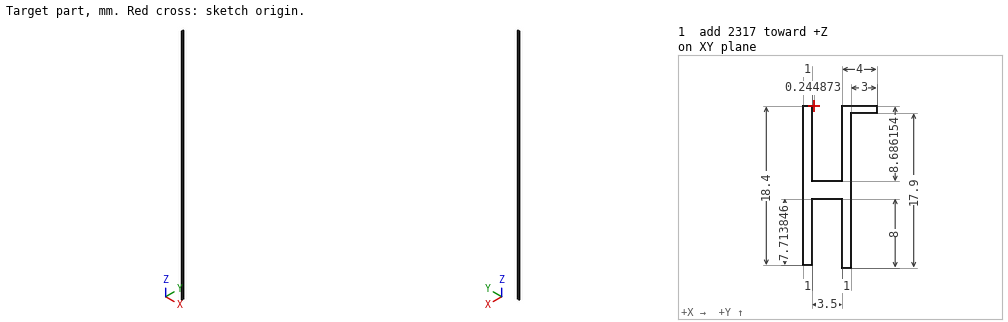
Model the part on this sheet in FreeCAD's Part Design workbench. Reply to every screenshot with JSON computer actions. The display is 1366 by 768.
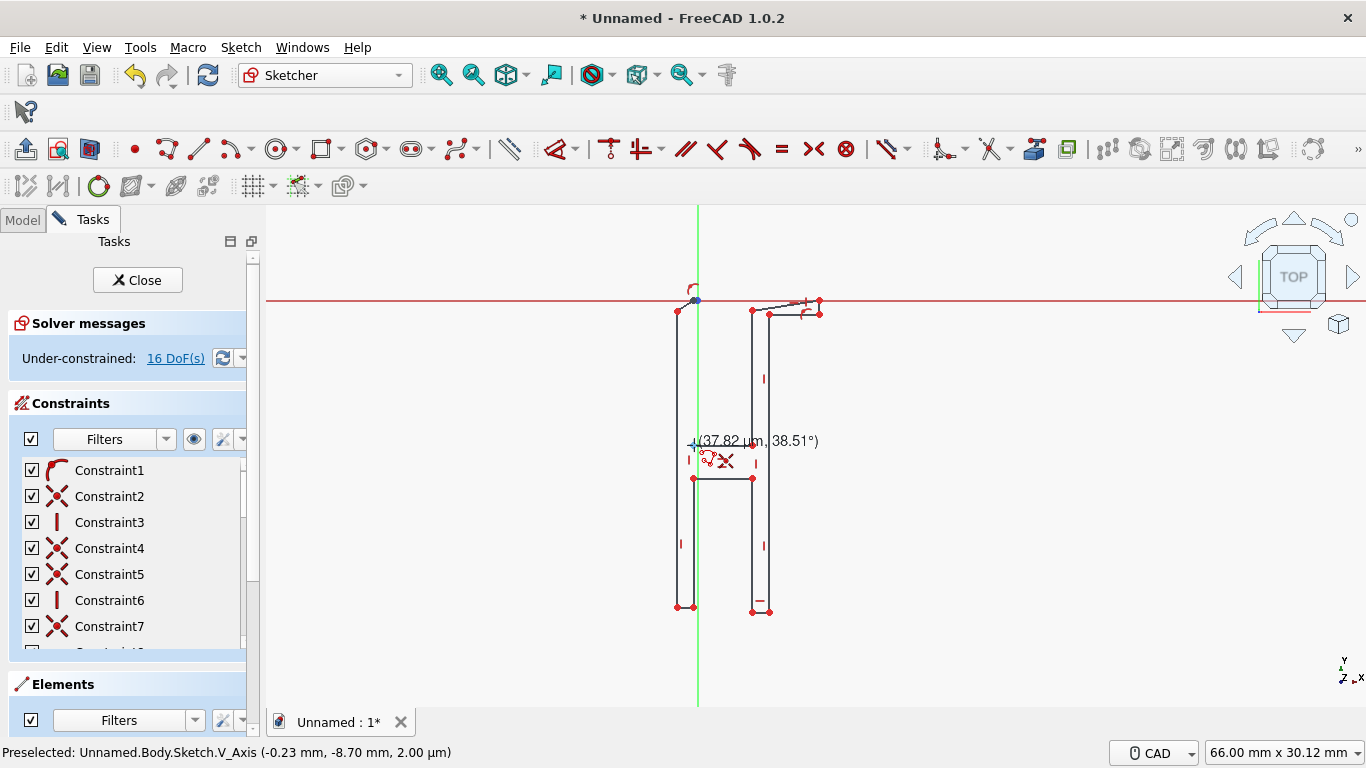
{"action": "scroll", "coordinate": [694, 301], "scroll_direction": "up", "scroll_amount": 7}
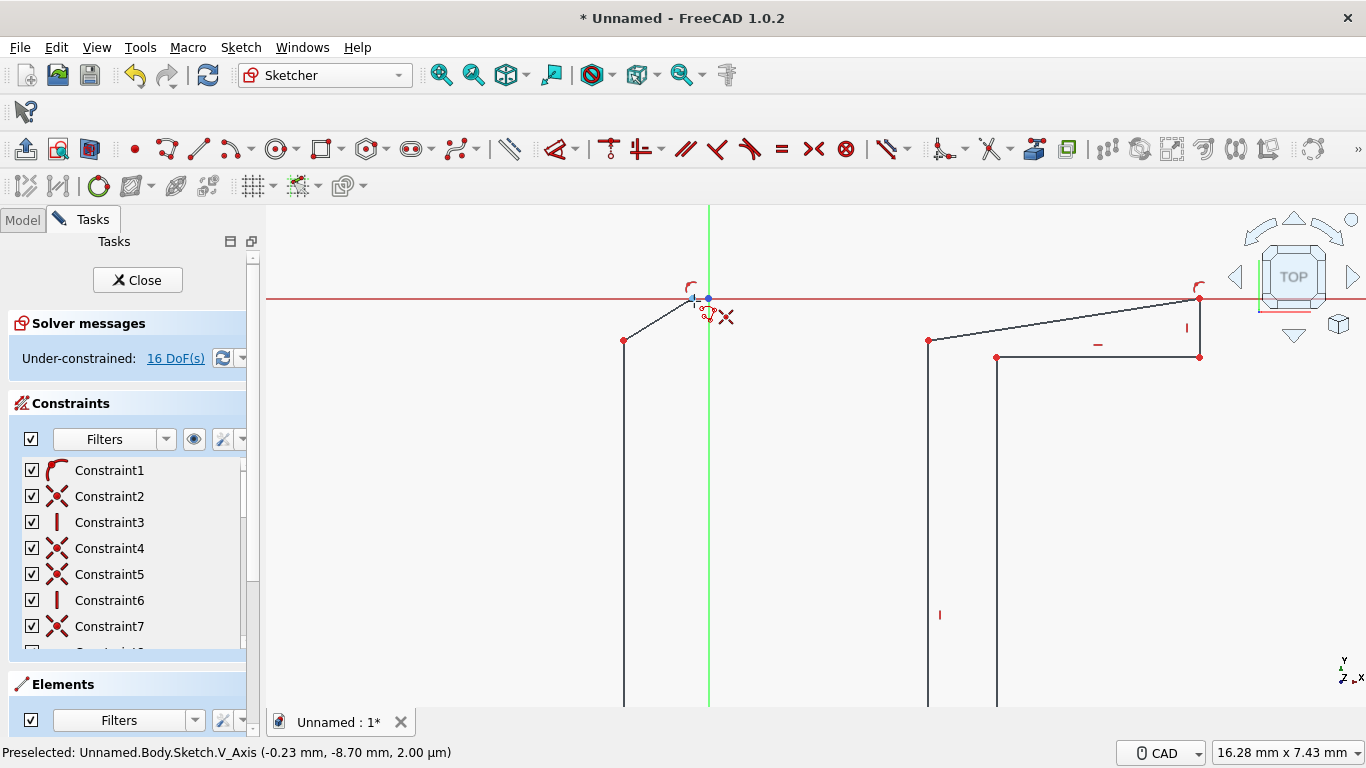
{"action": "left_click", "coordinate": [692, 299]}
{"action": "key", "text": "Escape"}
{"action": "key", "text": "Escape"}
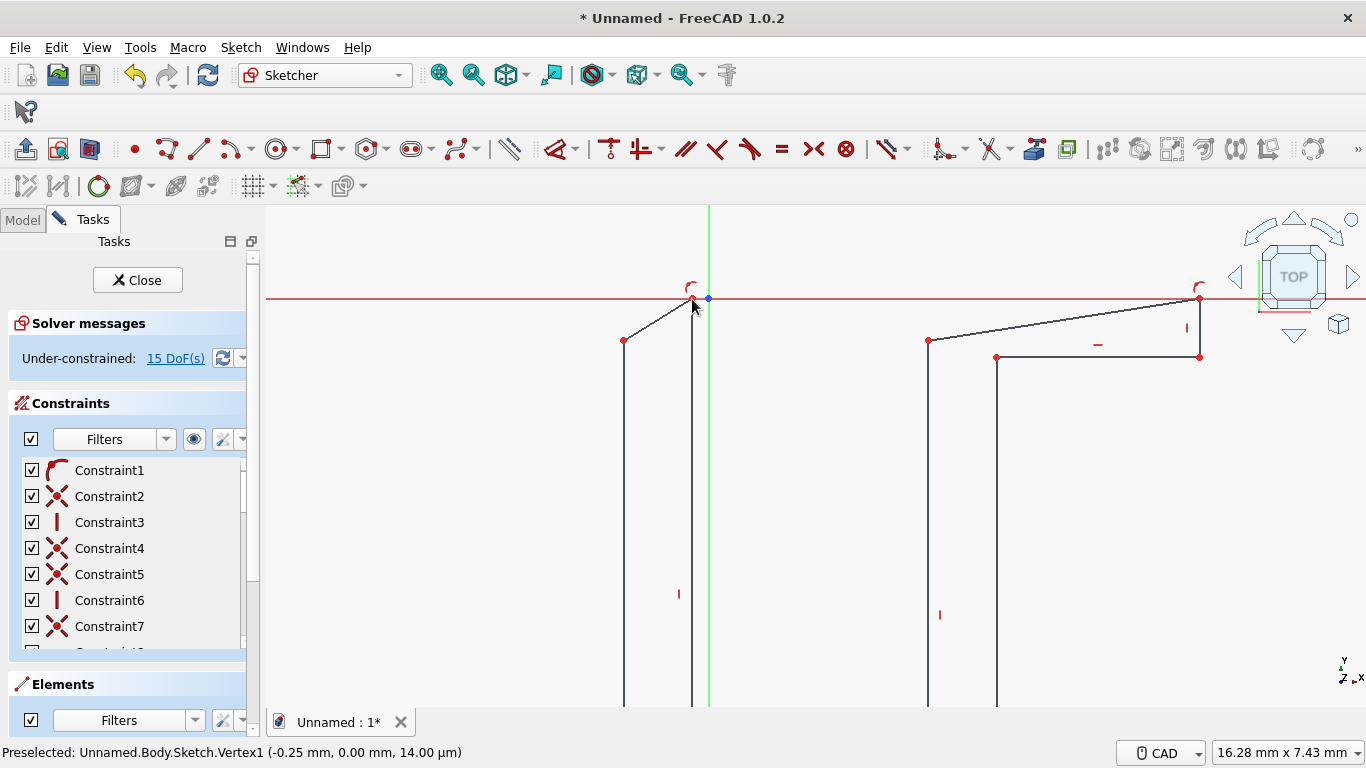
{"action": "left_click", "coordinate": [672, 311]}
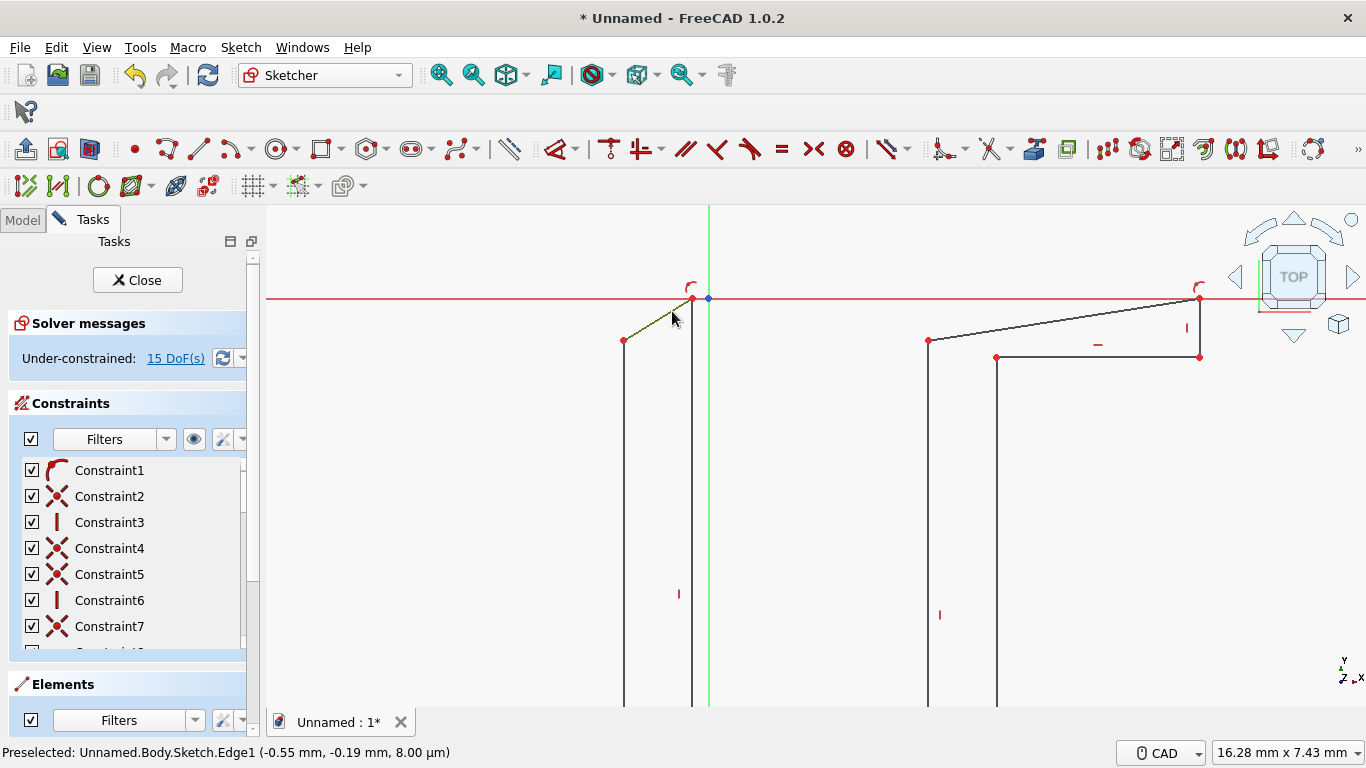
{"action": "key", "text": "h"}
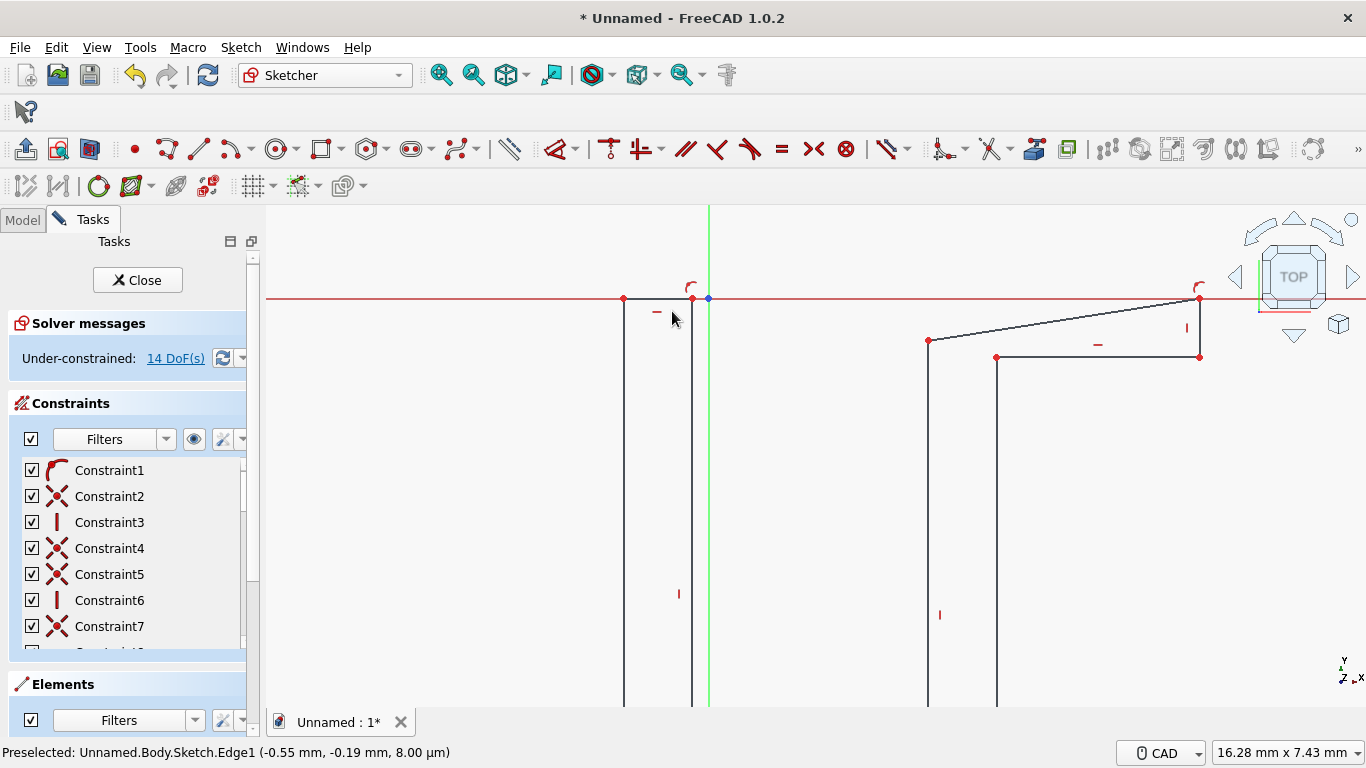
{"action": "scroll", "coordinate": [694, 301], "scroll_direction": "down", "scroll_amount": 7}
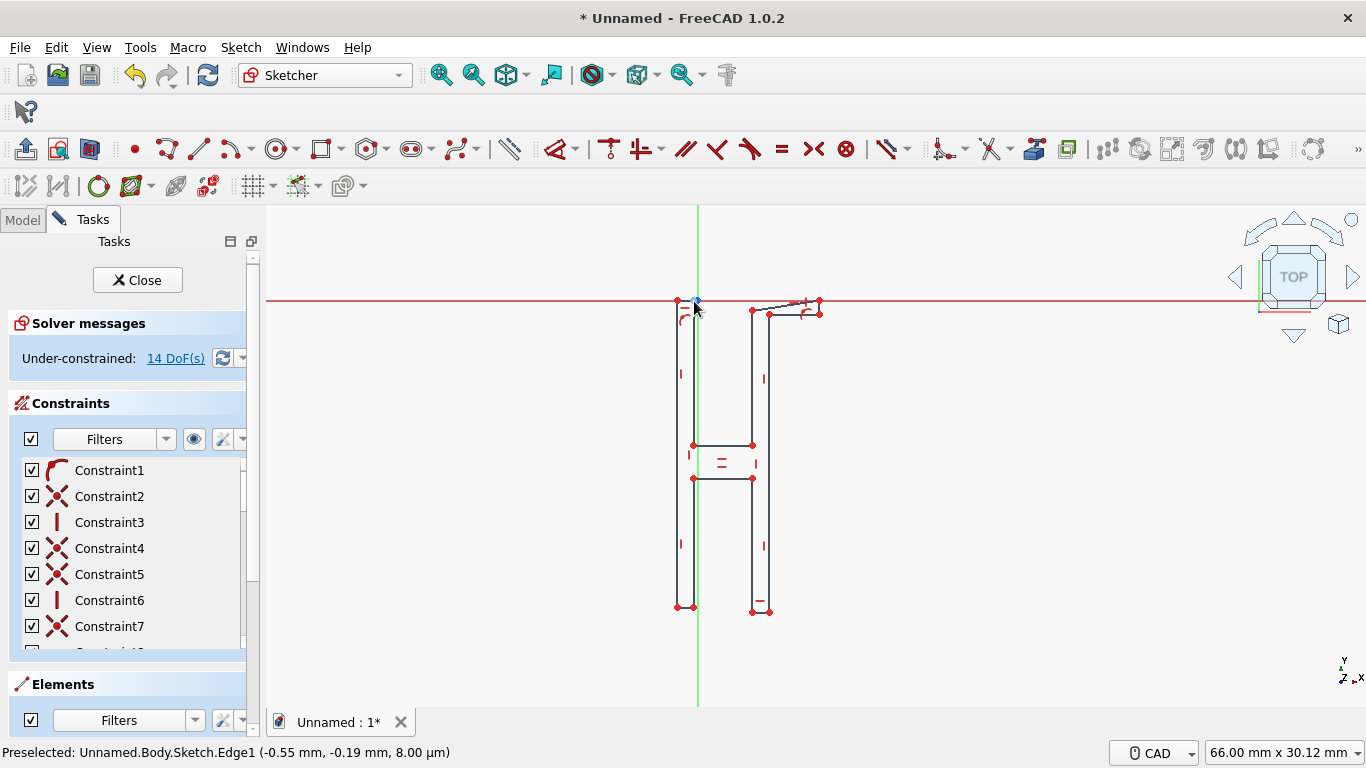
{"action": "scroll", "coordinate": [682, 608], "scroll_direction": "up", "scroll_amount": 6}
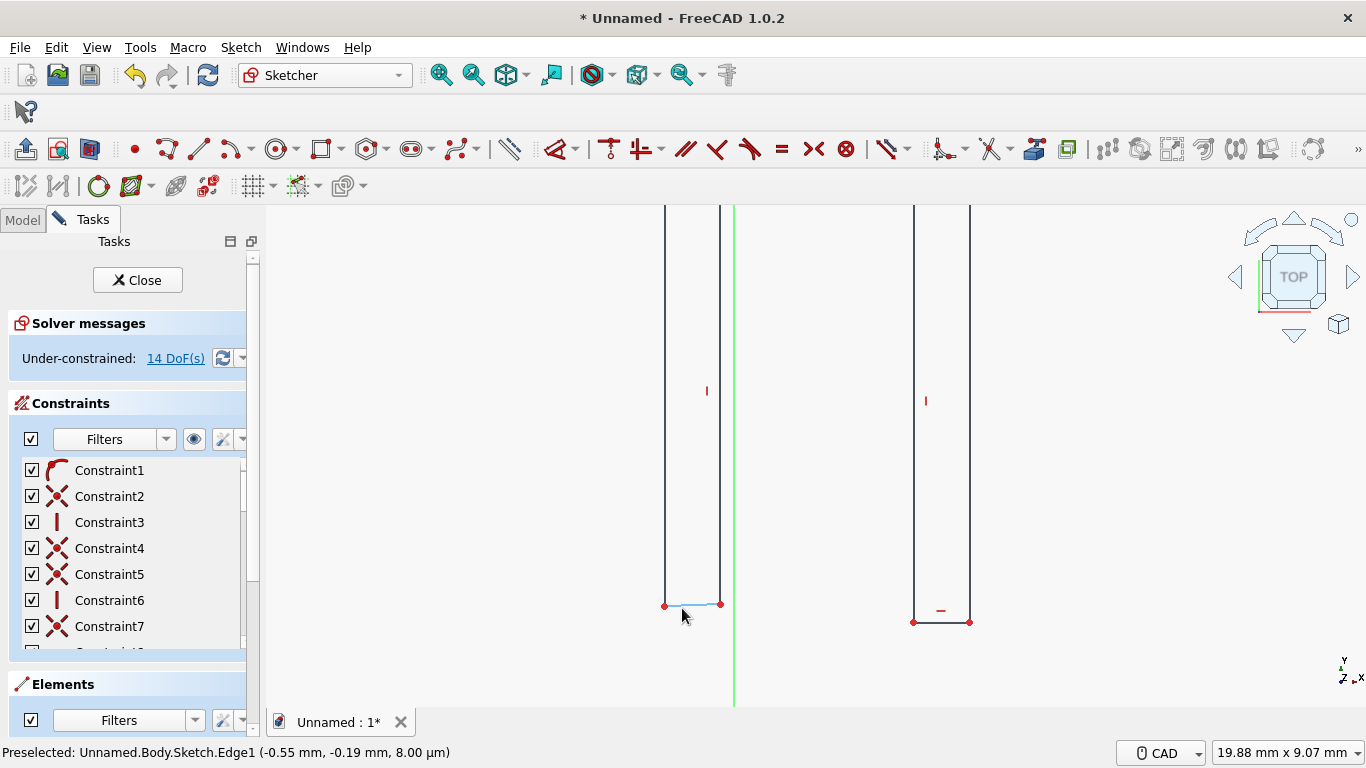
{"action": "left_click", "coordinate": [681, 605]}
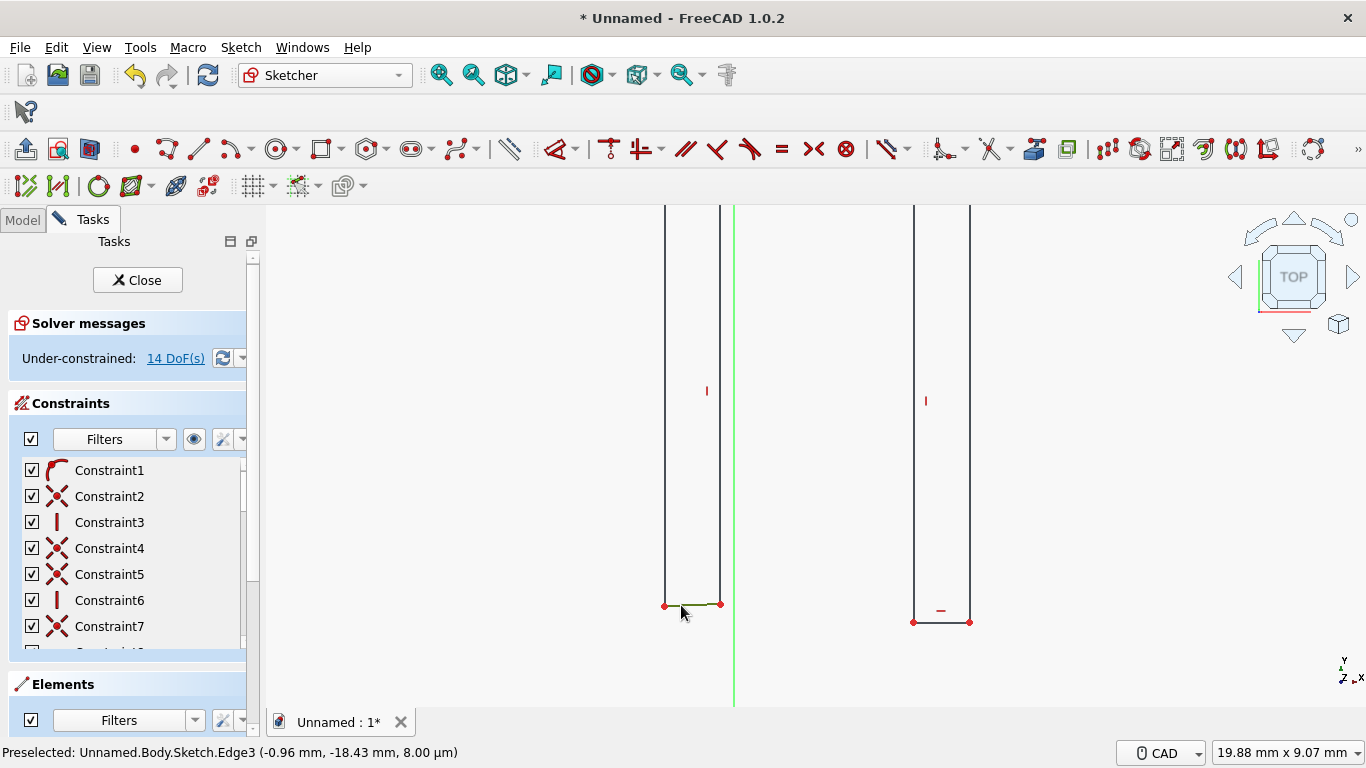
{"action": "key", "text": "h"}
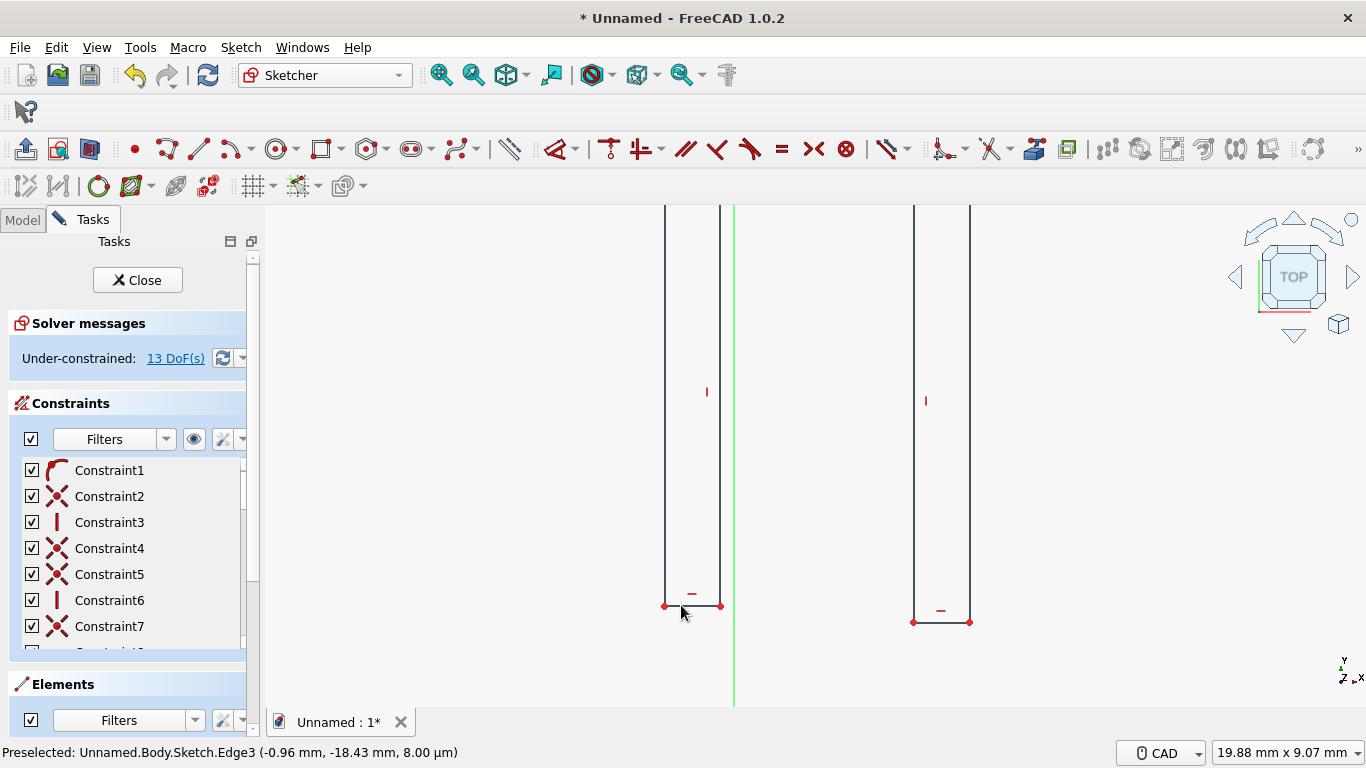
{"action": "scroll", "coordinate": [682, 608], "scroll_direction": "down", "scroll_amount": 6}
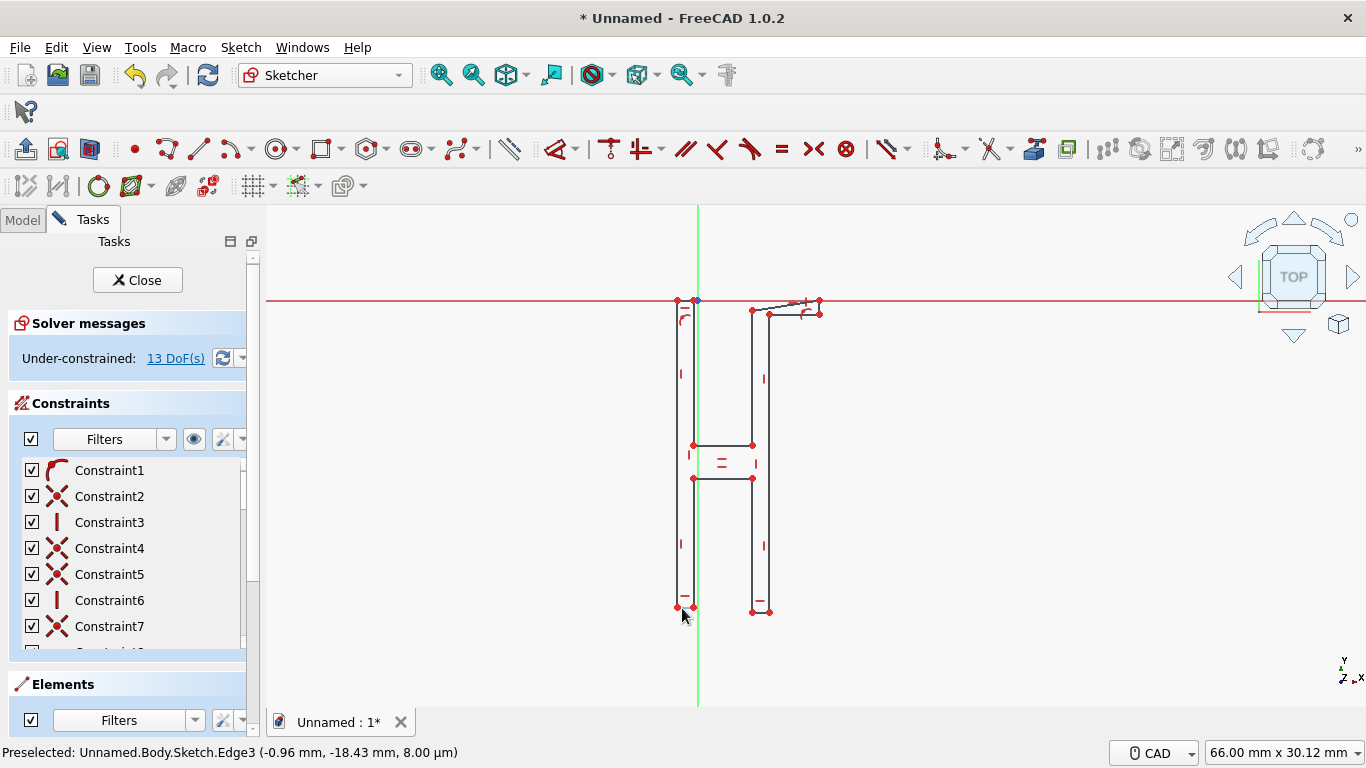
{"action": "scroll", "coordinate": [799, 304], "scroll_direction": "up", "scroll_amount": 8}